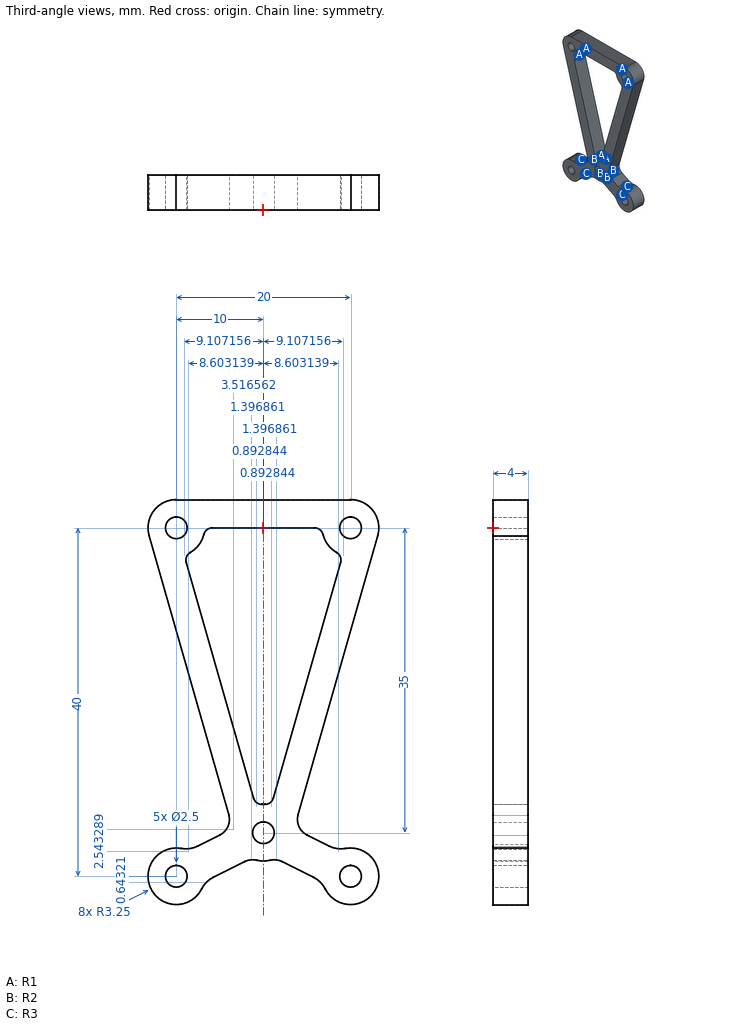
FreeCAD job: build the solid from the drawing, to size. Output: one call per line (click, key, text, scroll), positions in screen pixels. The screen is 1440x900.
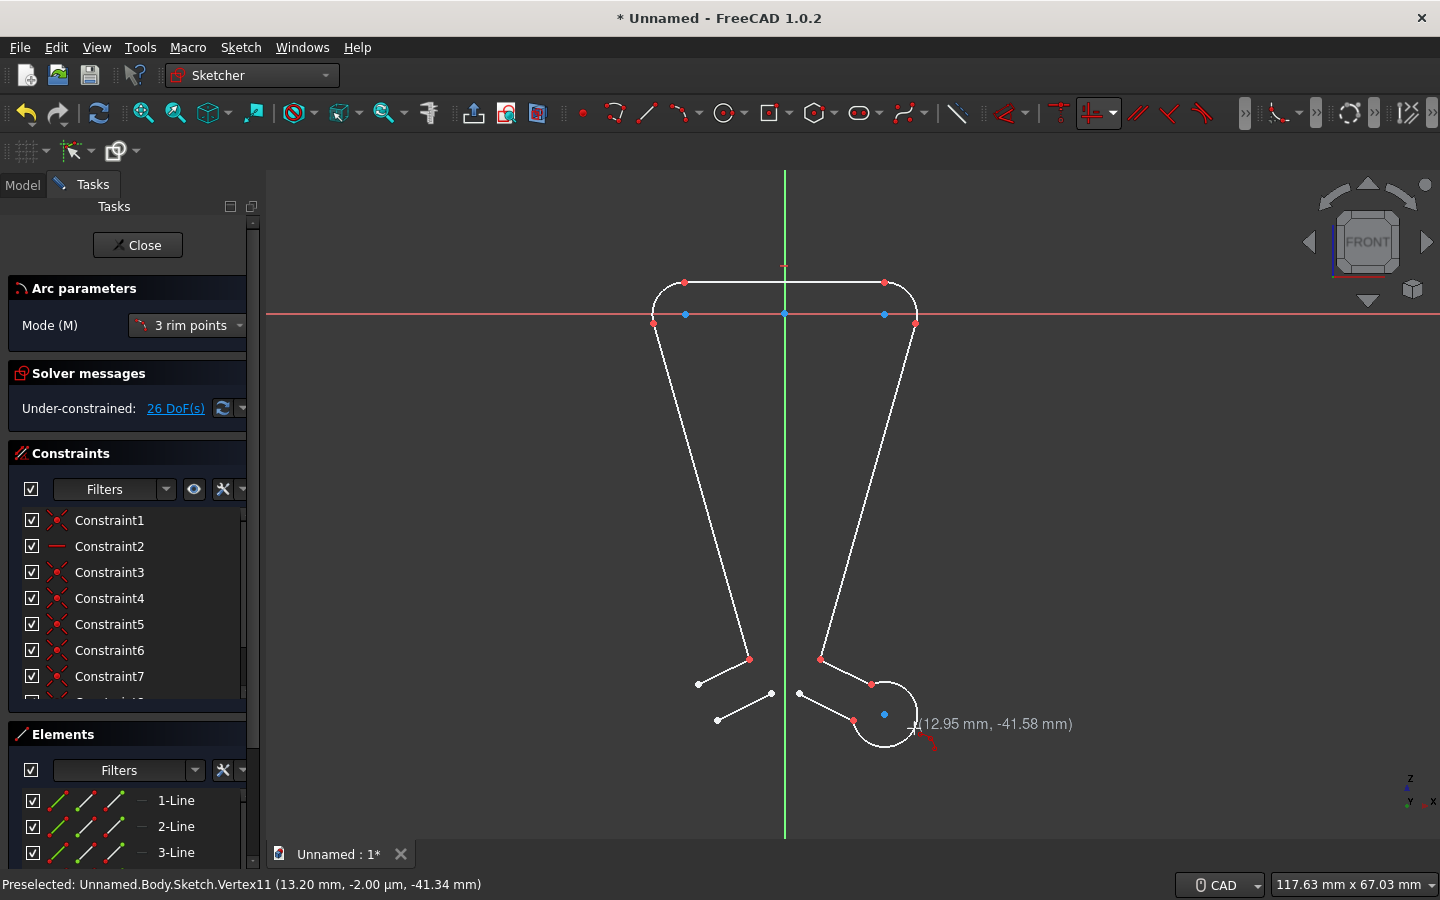
click(799, 694)
click(771, 694)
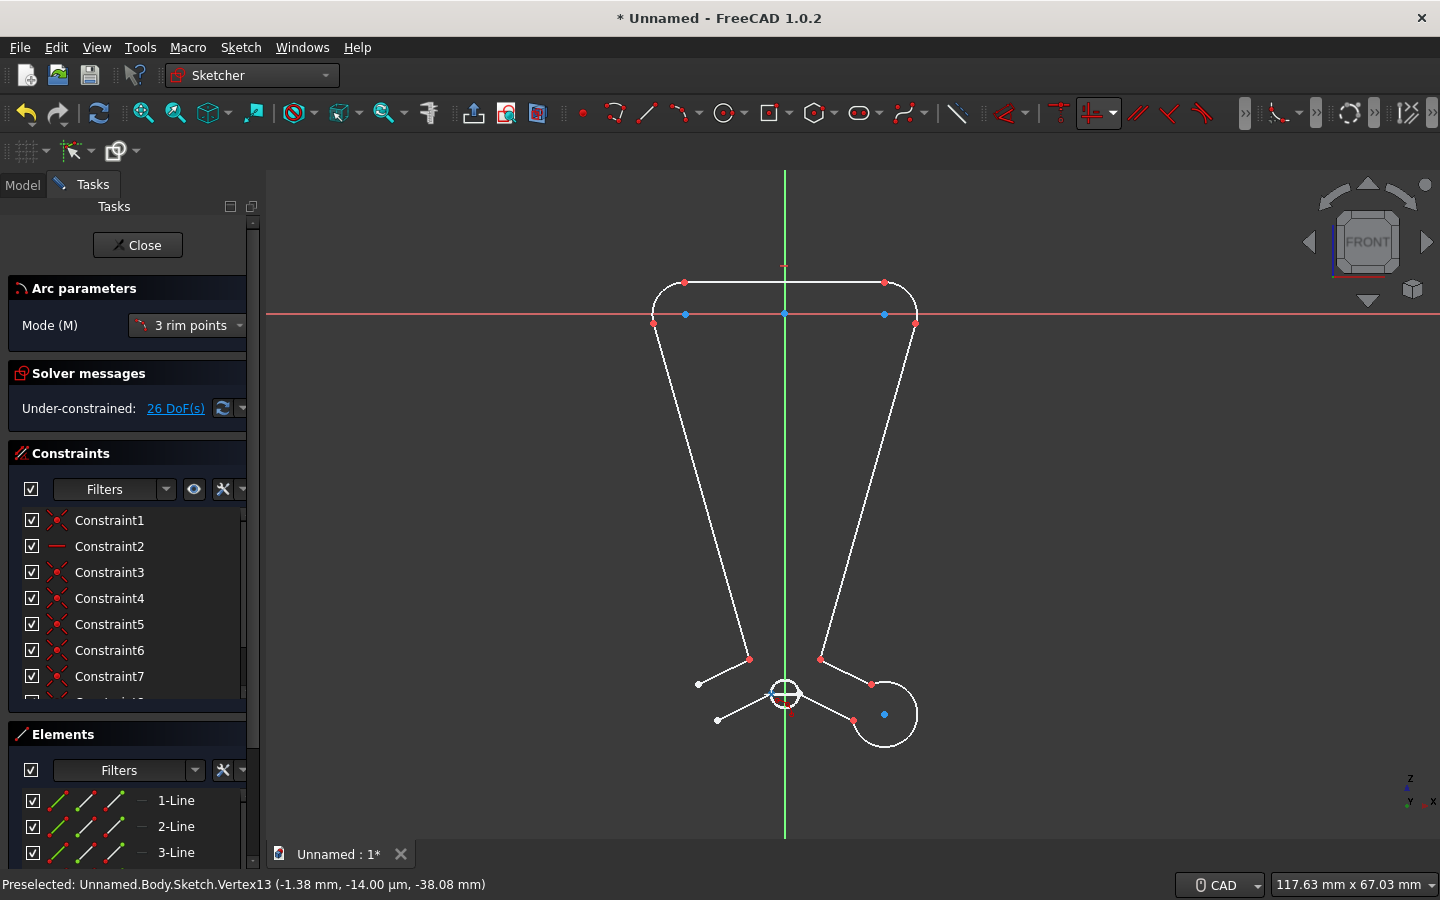
scroll(788, 696, up, 9)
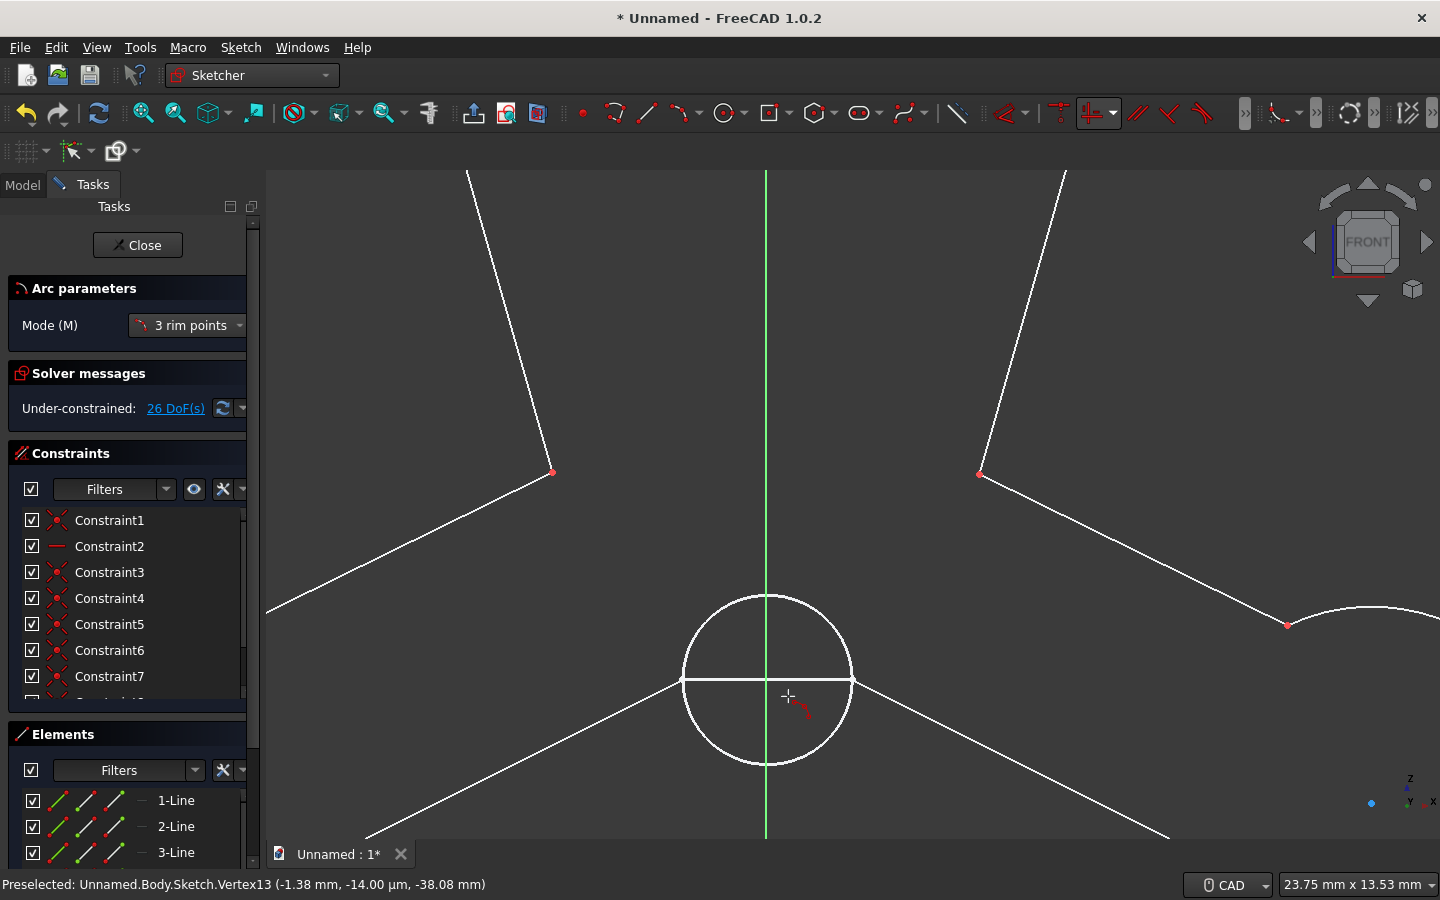
click(784, 690)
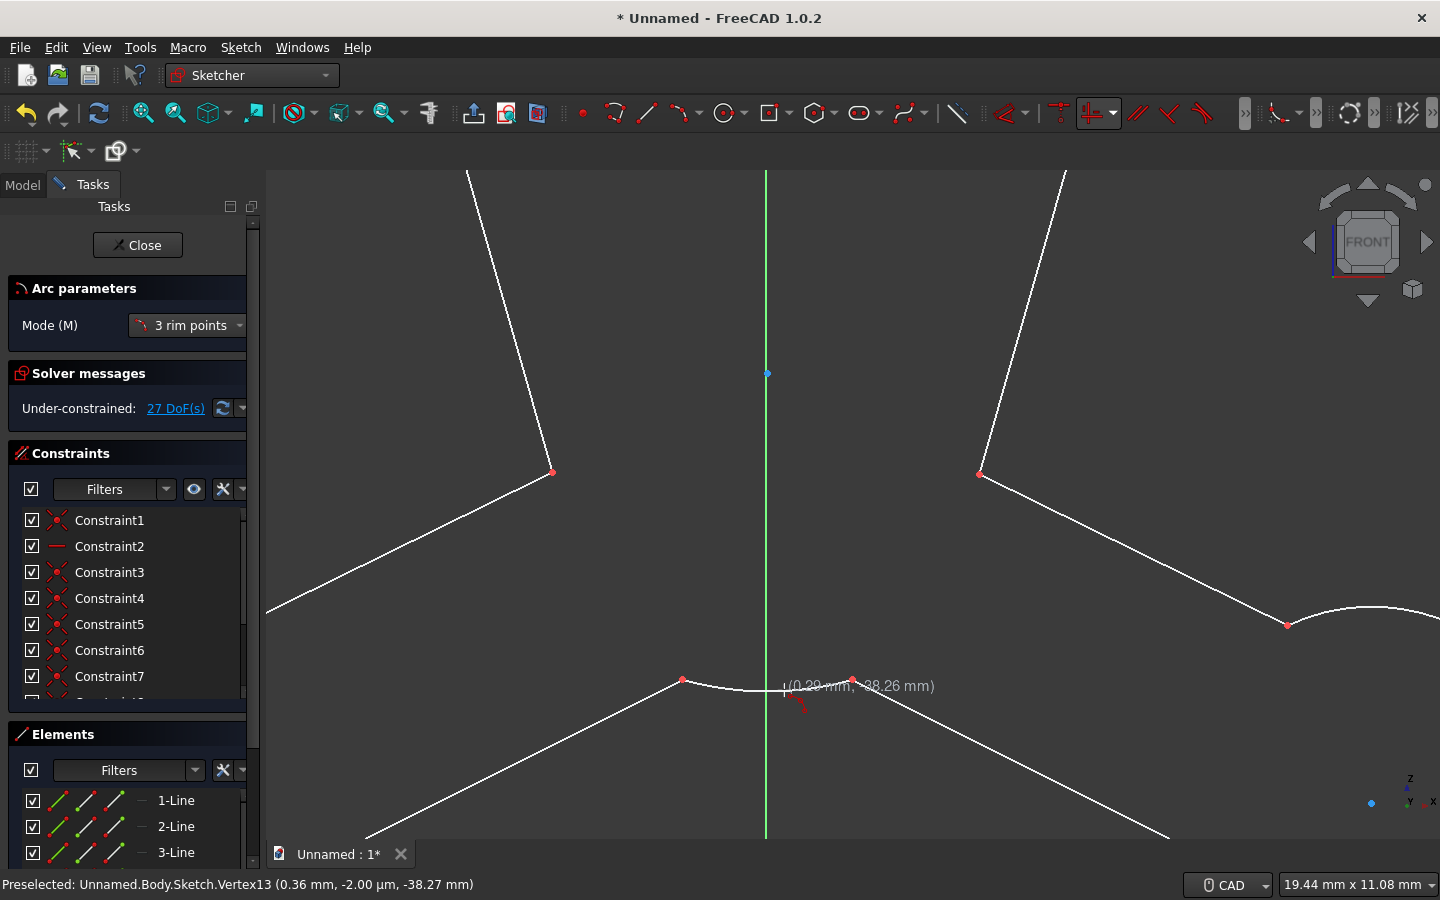
scroll(788, 697, down, 9)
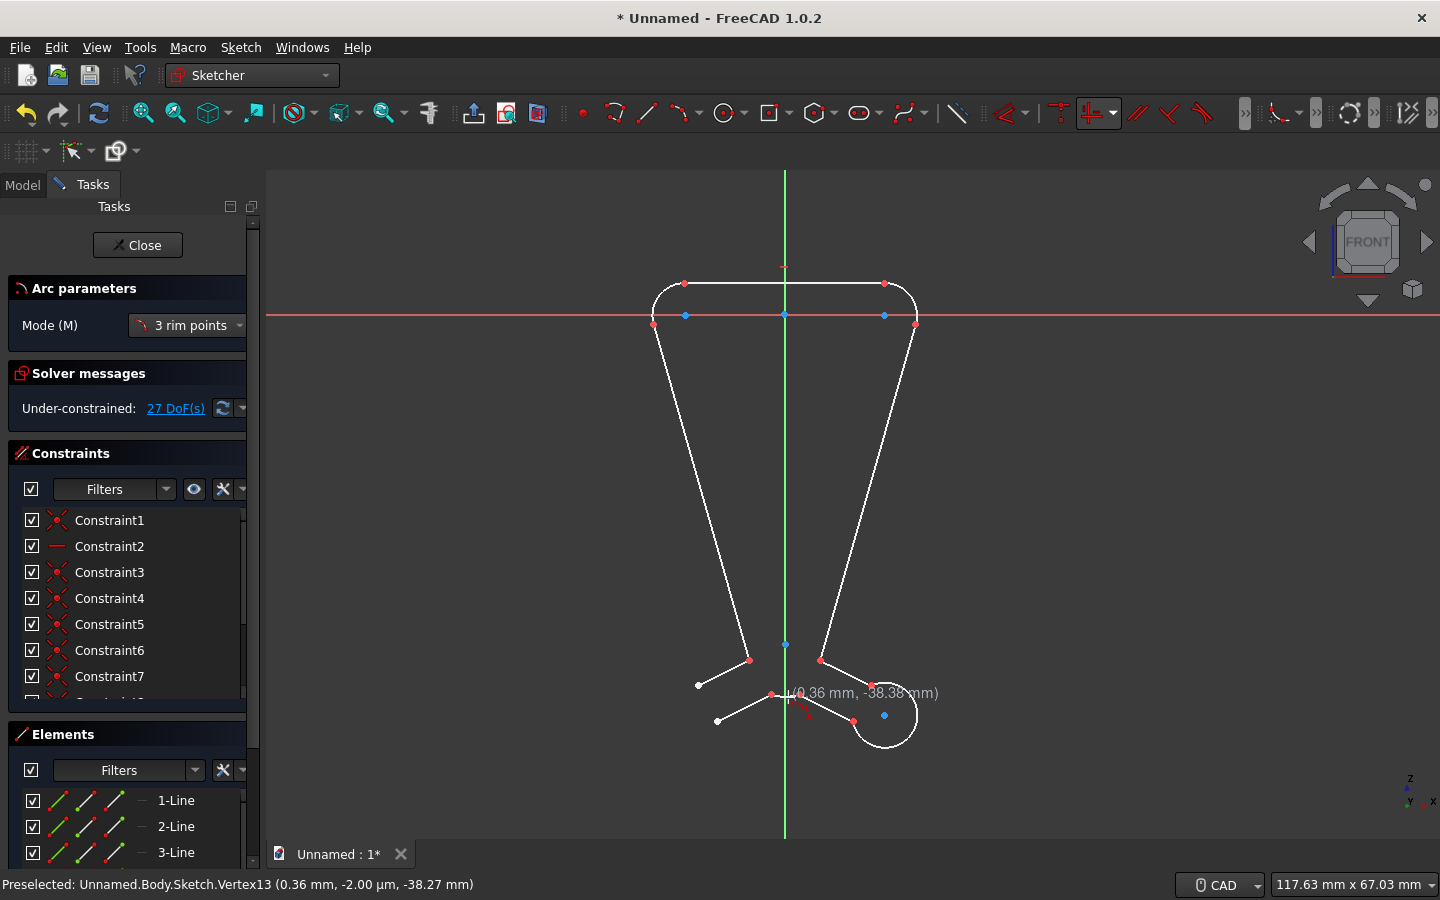
click(717, 722)
click(698, 686)
click(656, 729)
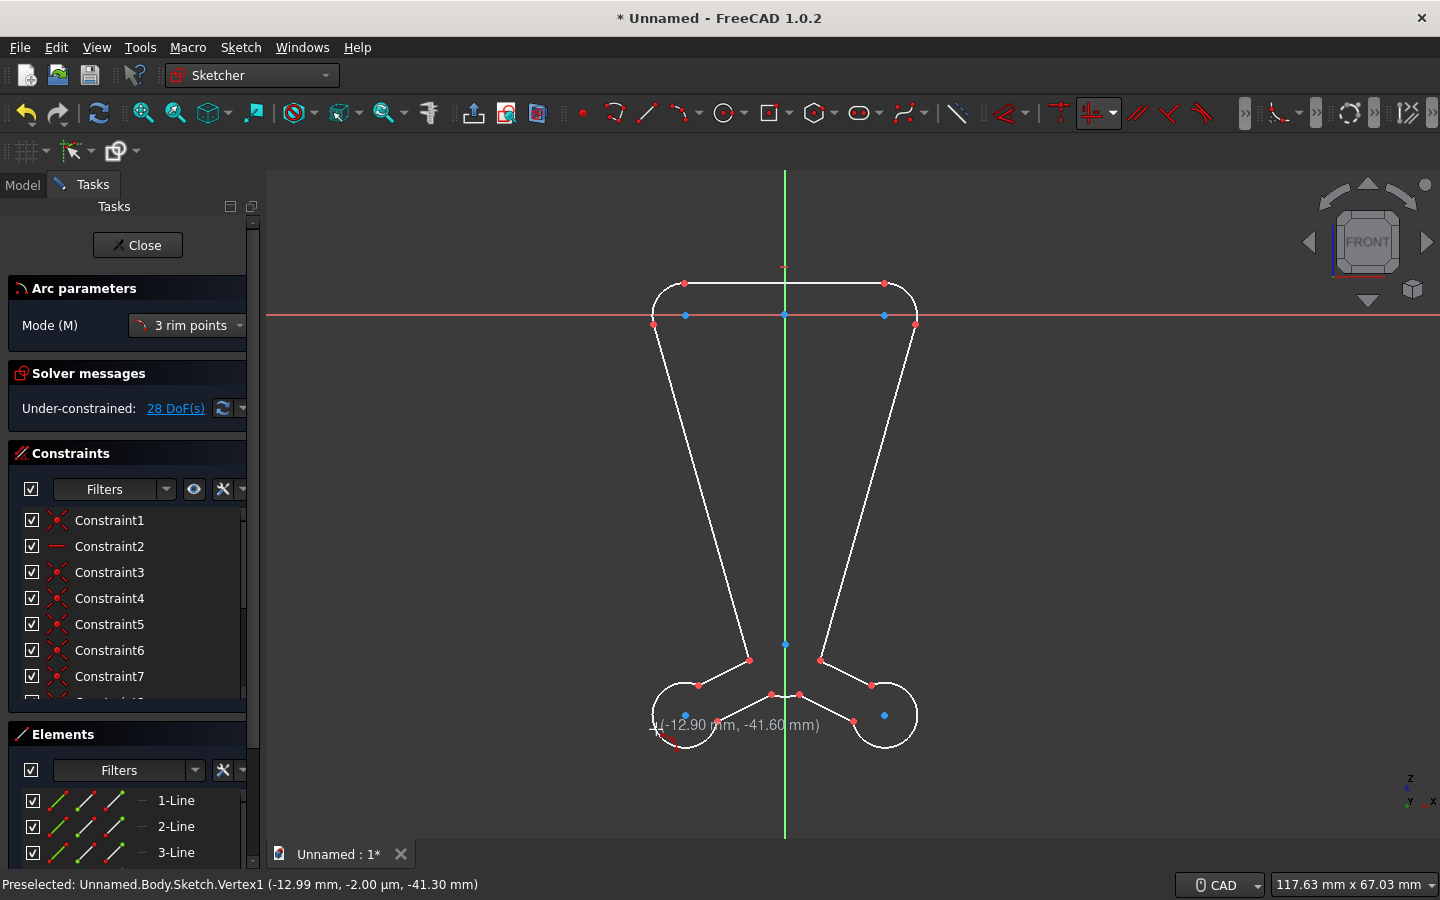
click(648, 114)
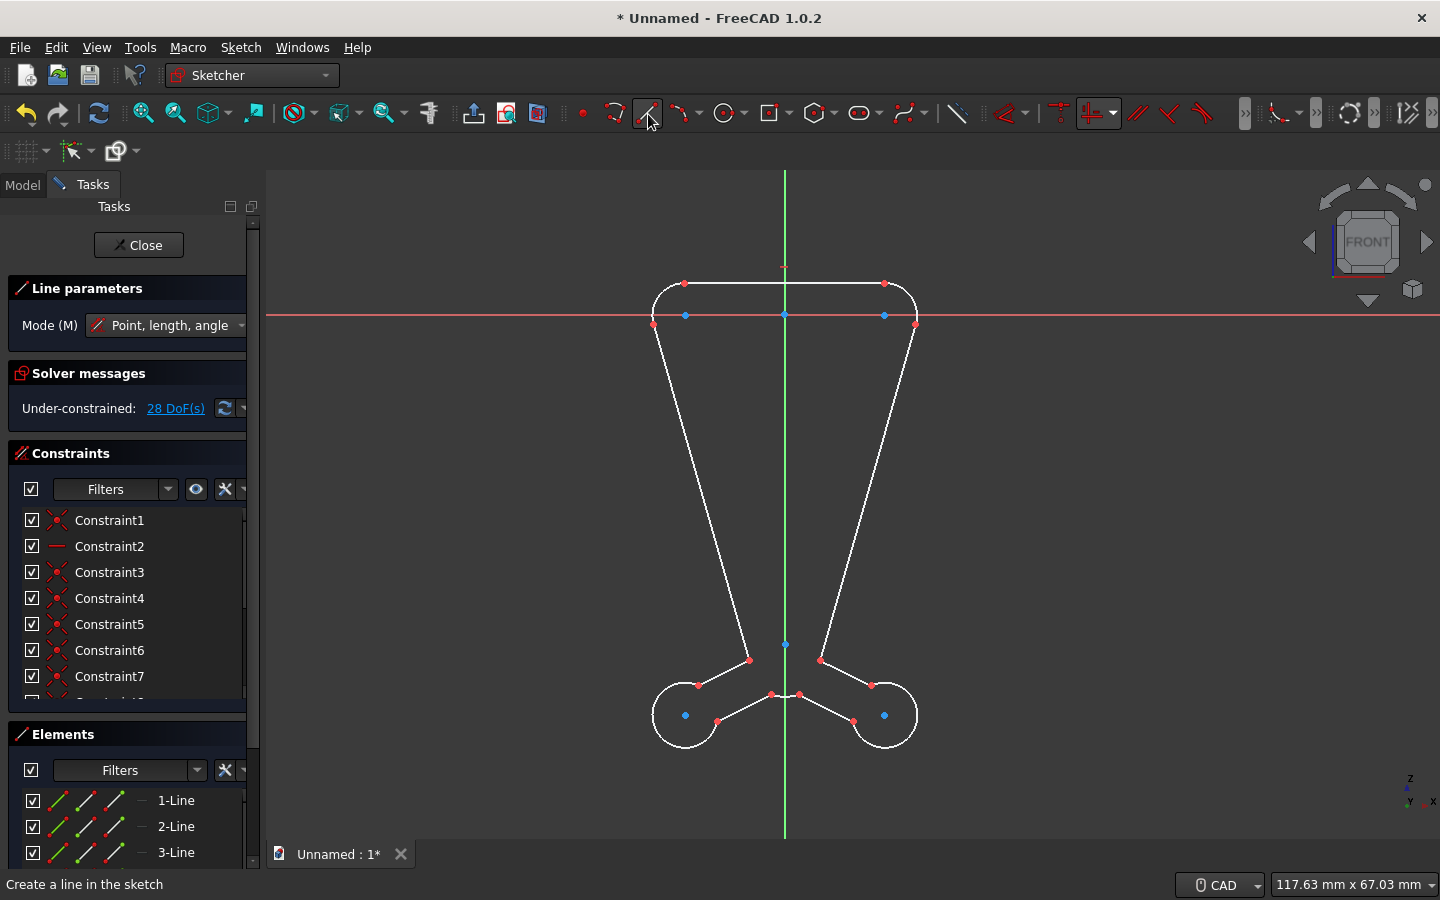
scroll(794, 633, up, 3)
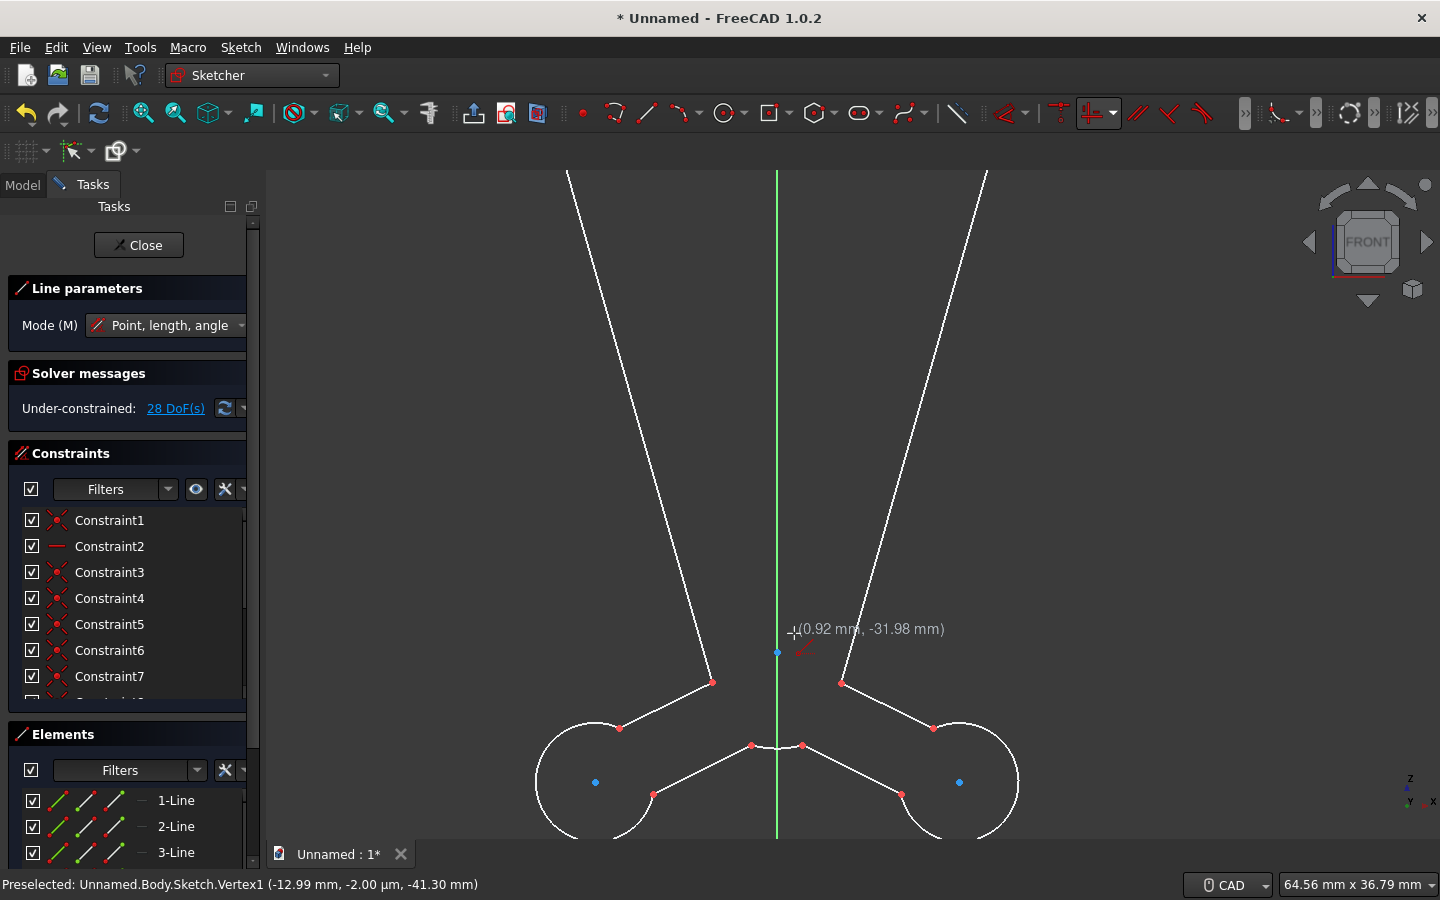
click(793, 632)